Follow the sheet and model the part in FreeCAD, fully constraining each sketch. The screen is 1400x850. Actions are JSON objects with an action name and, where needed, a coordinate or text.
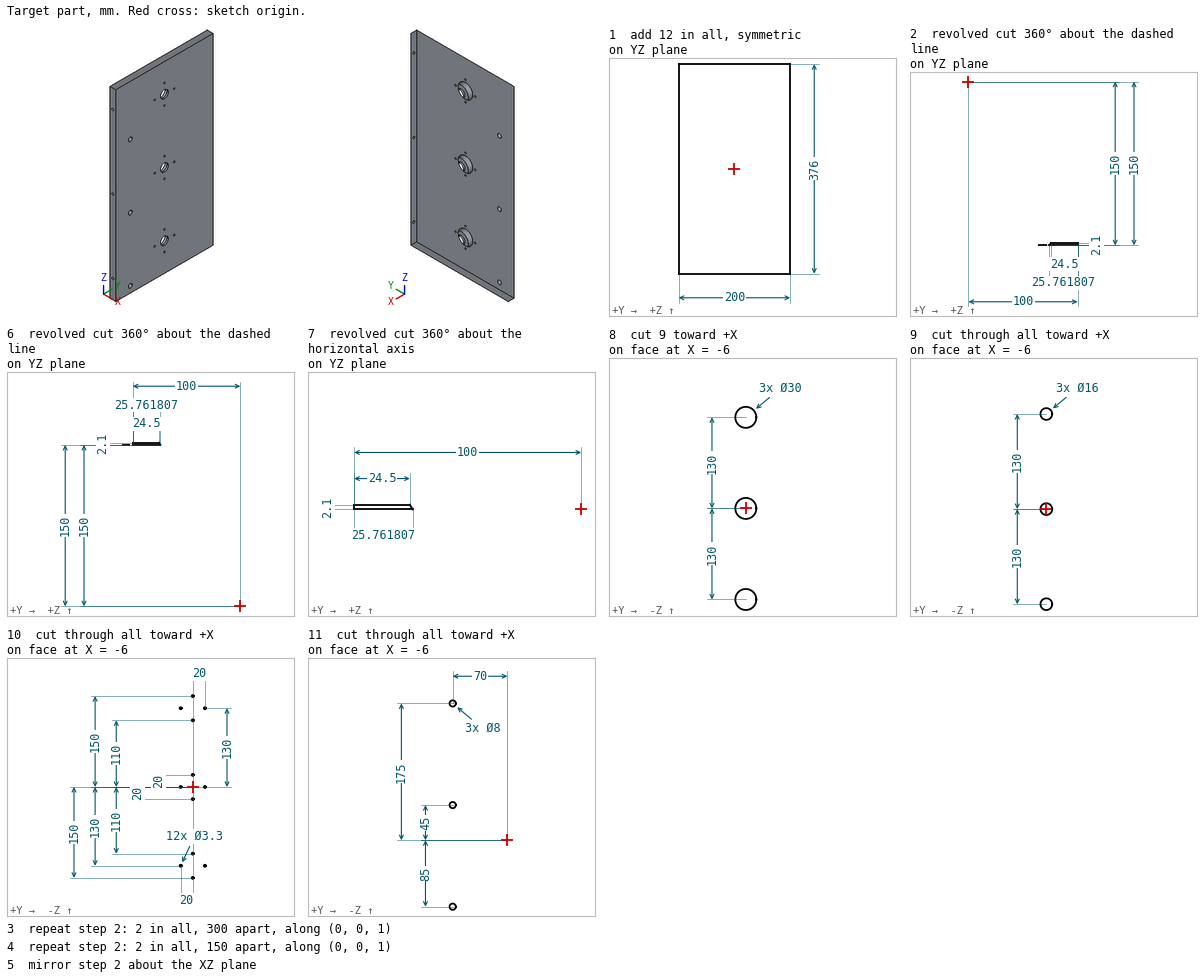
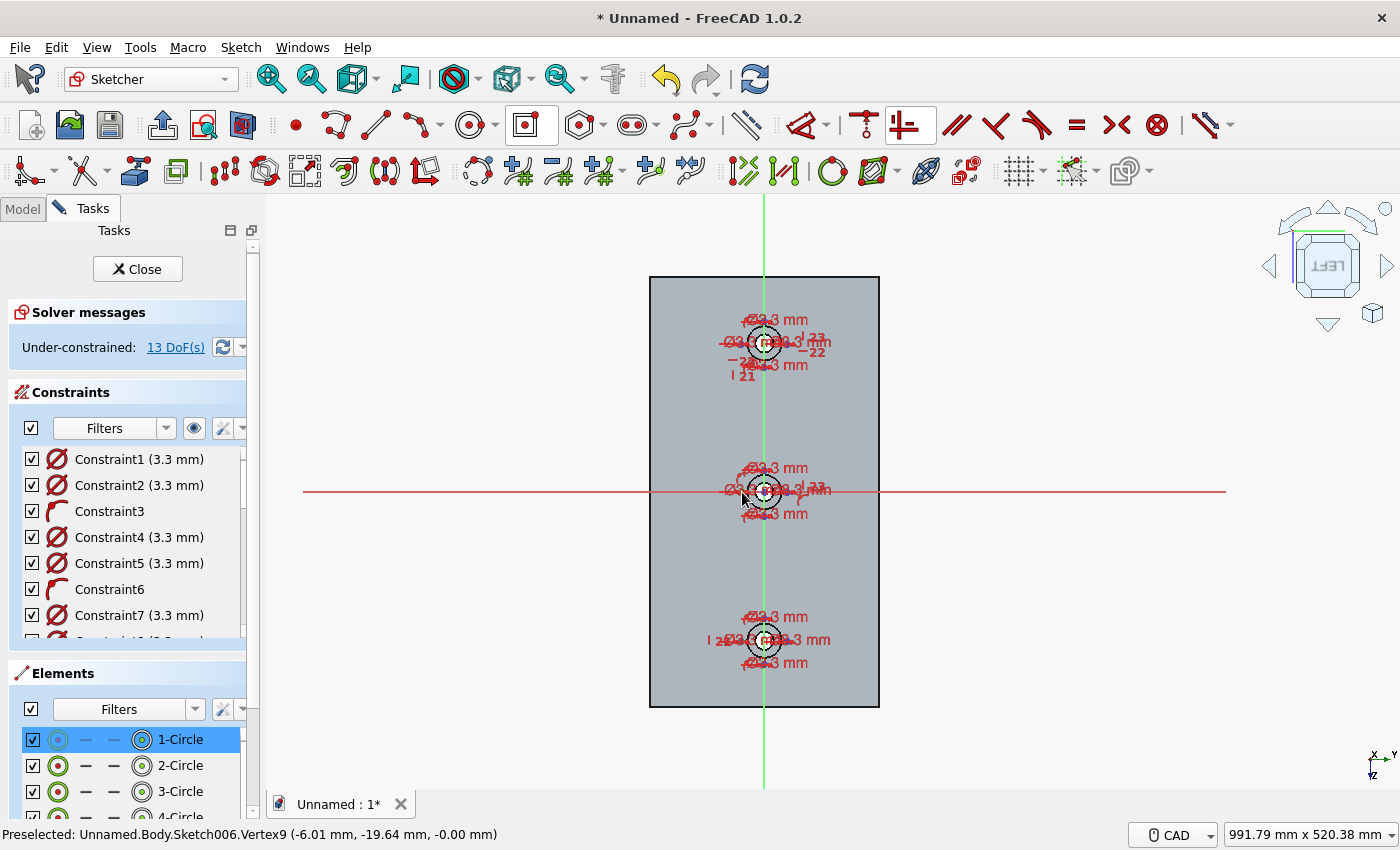
{"action": "key", "text": "v"}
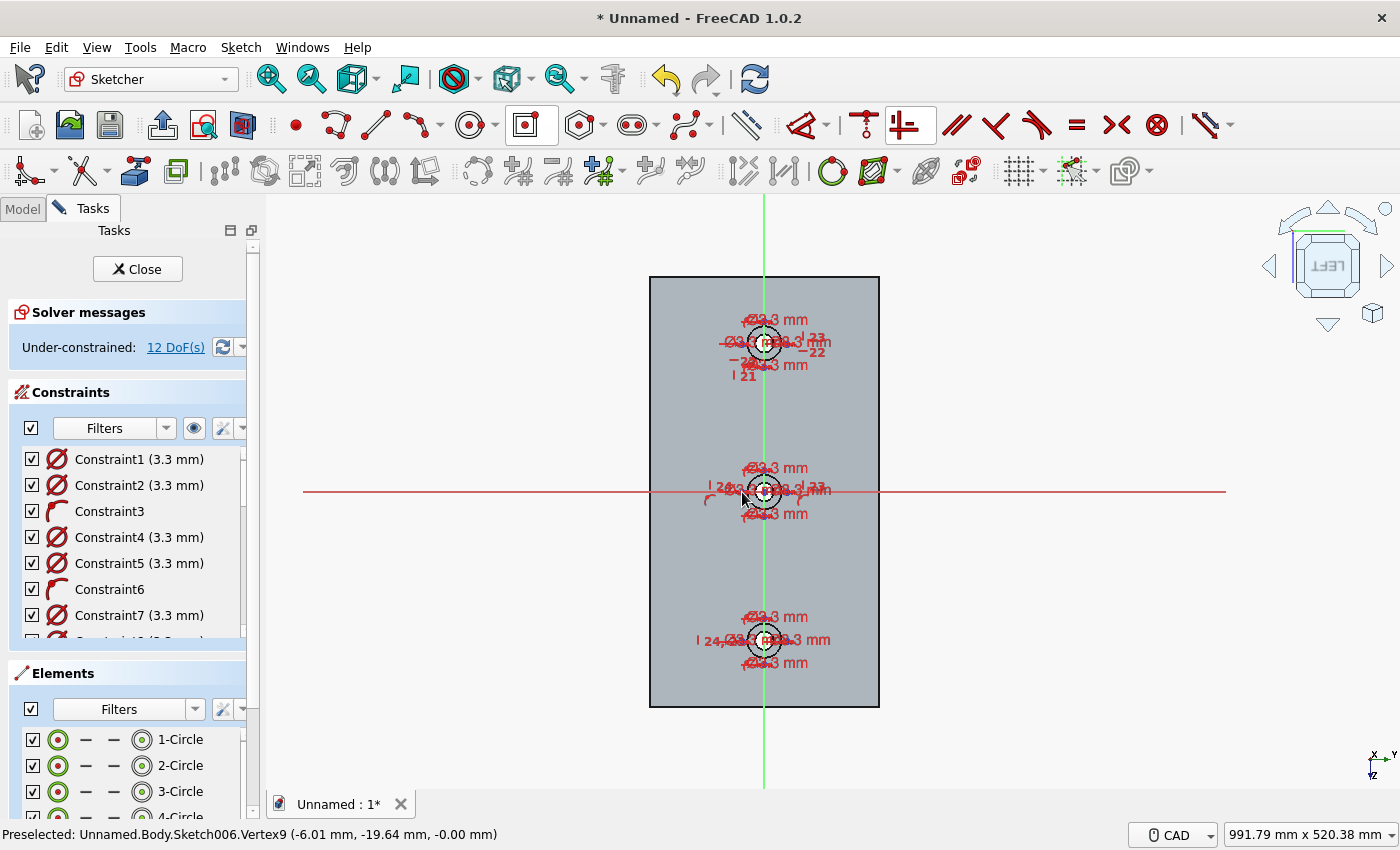
{"action": "left_click", "coordinate": [788, 492]}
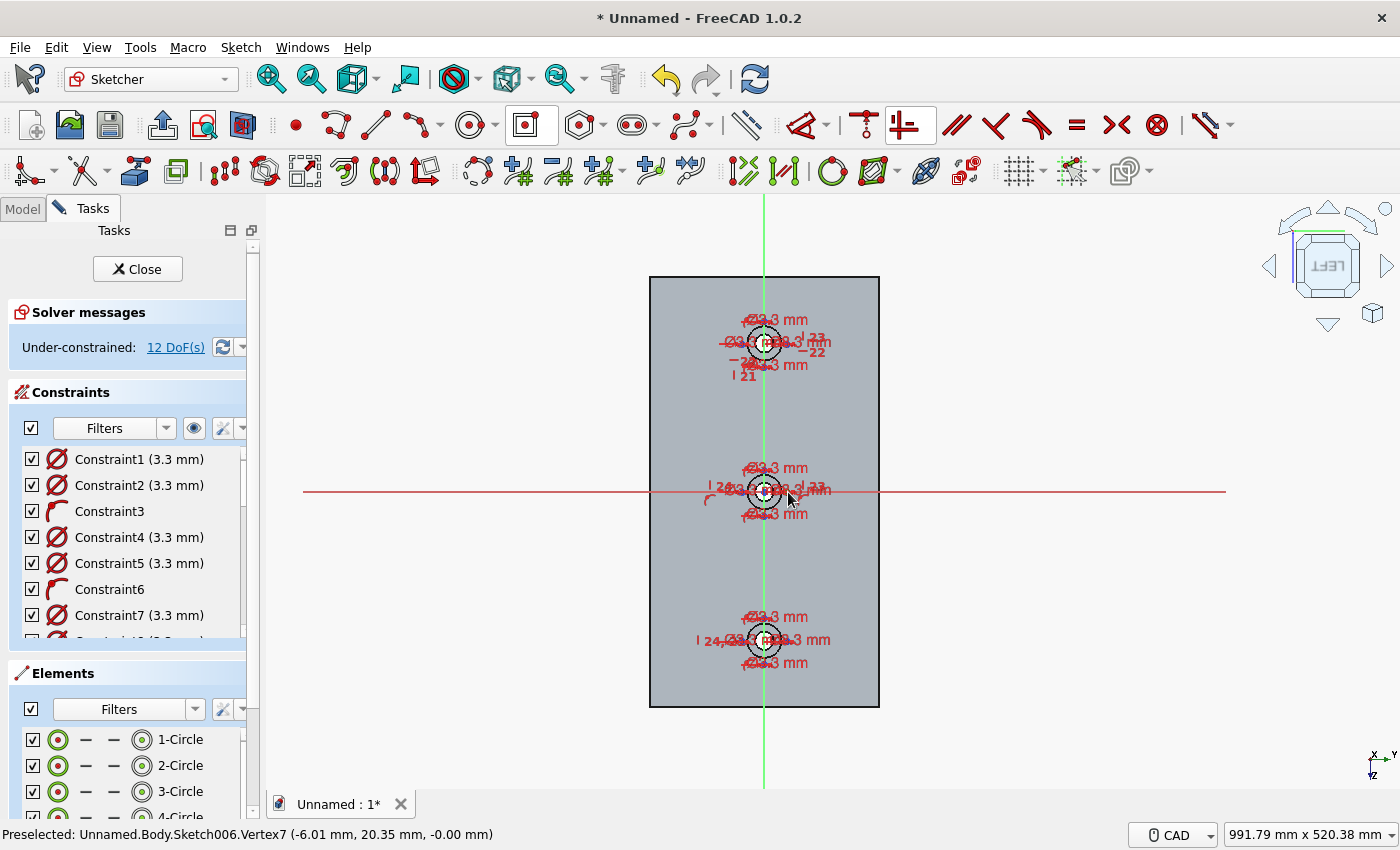
{"action": "left_click", "coordinate": [787, 642]}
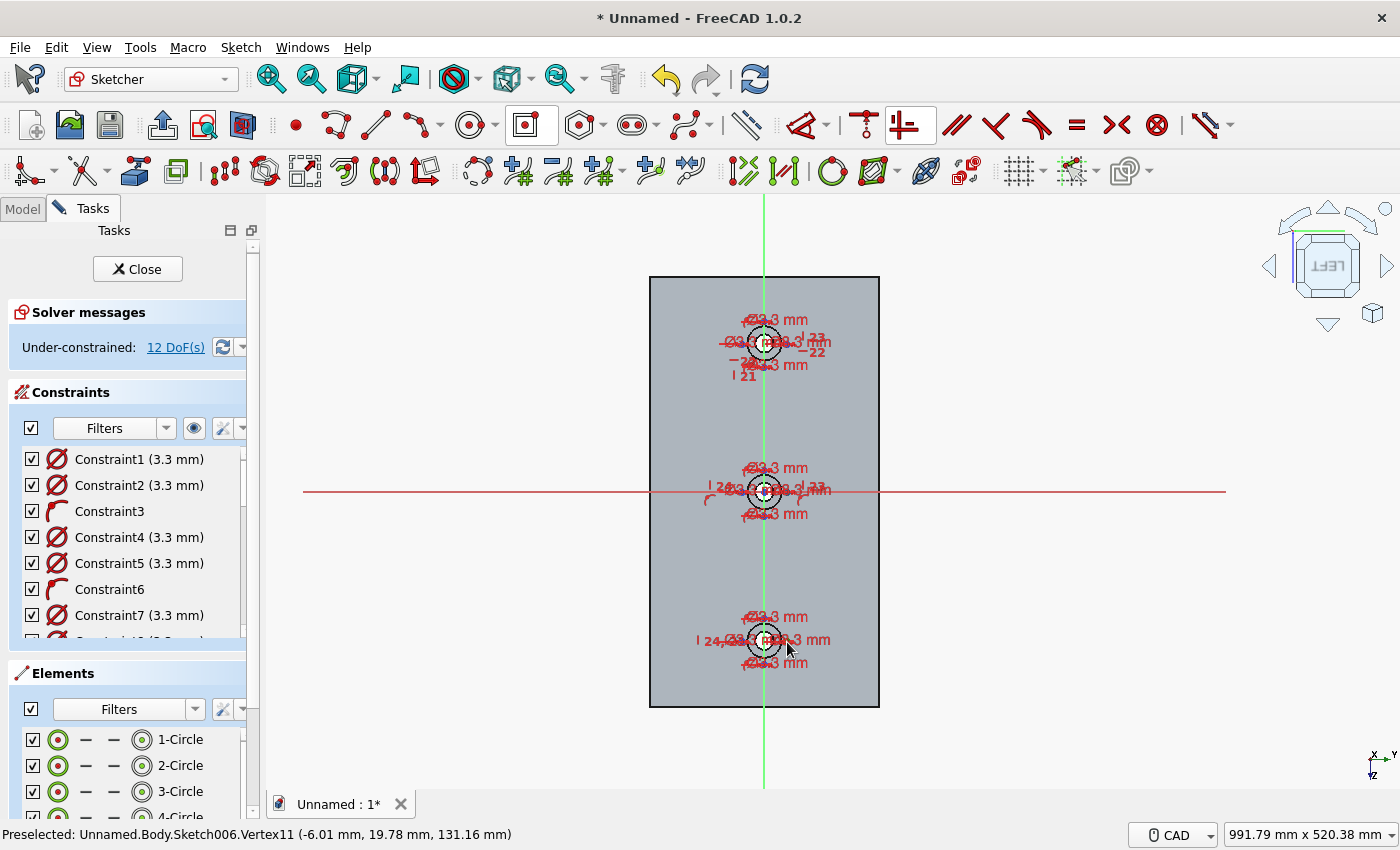
{"action": "key", "text": "v"}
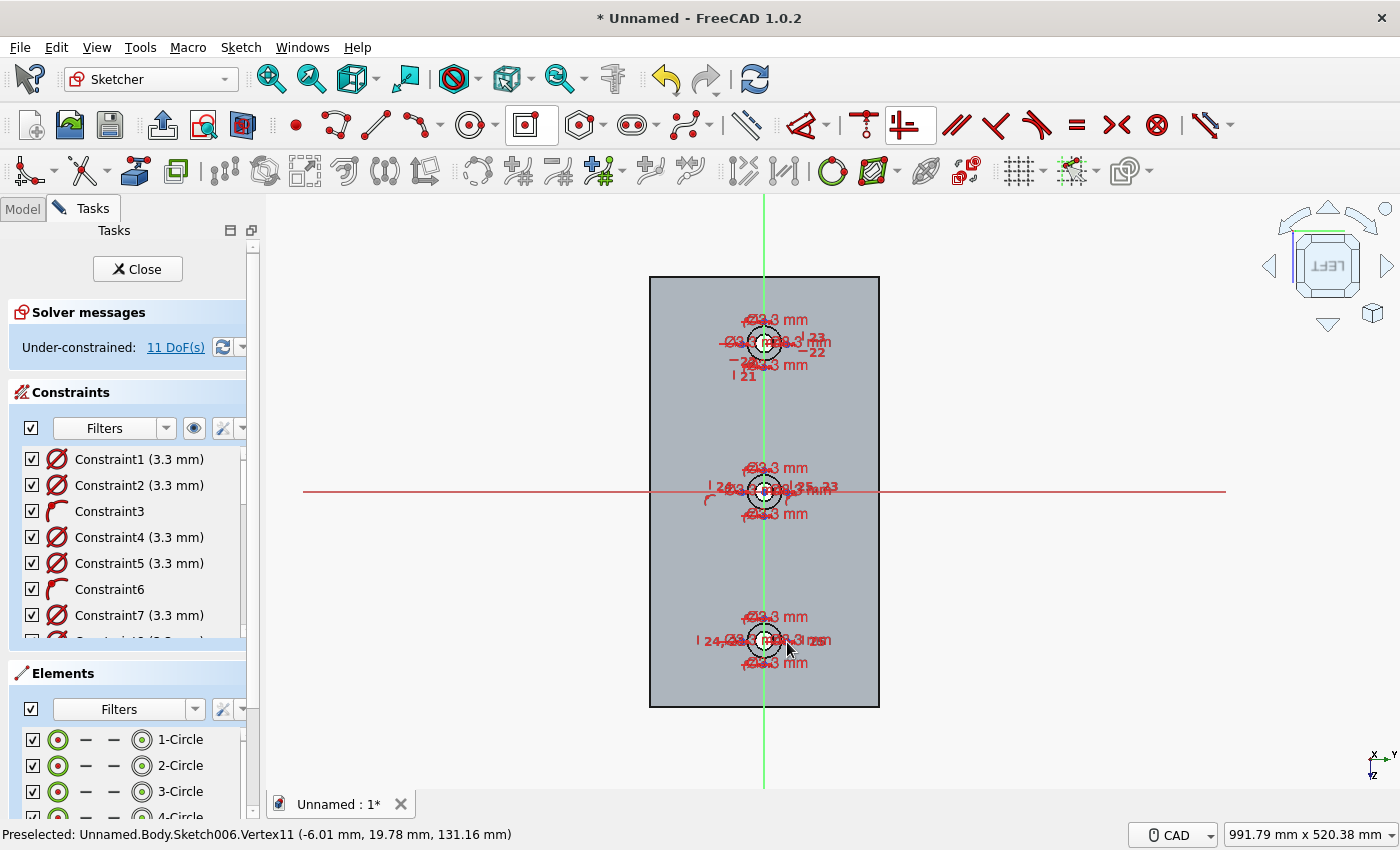
{"action": "left_click", "coordinate": [742, 642]}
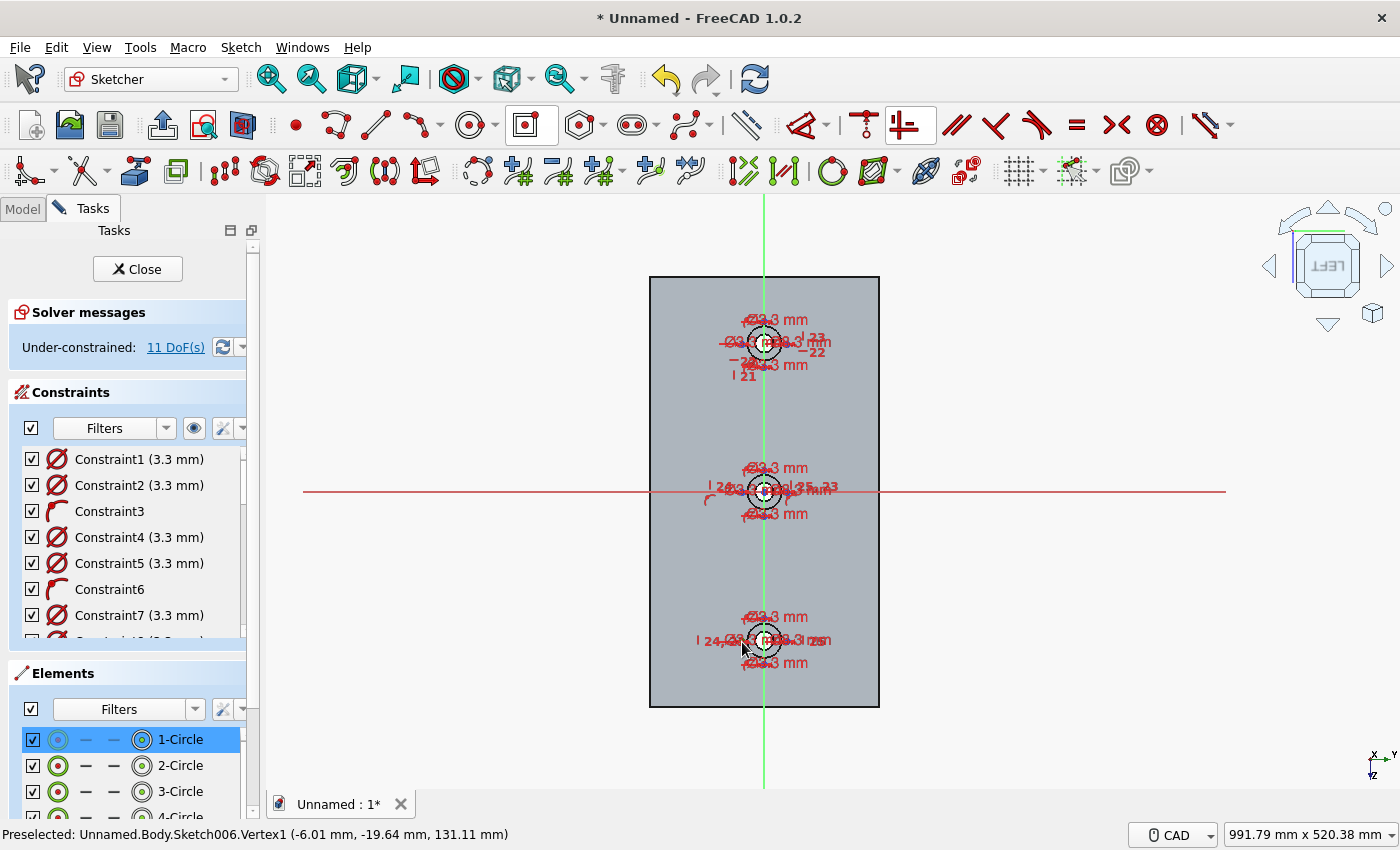
{"action": "left_click", "coordinate": [788, 642]}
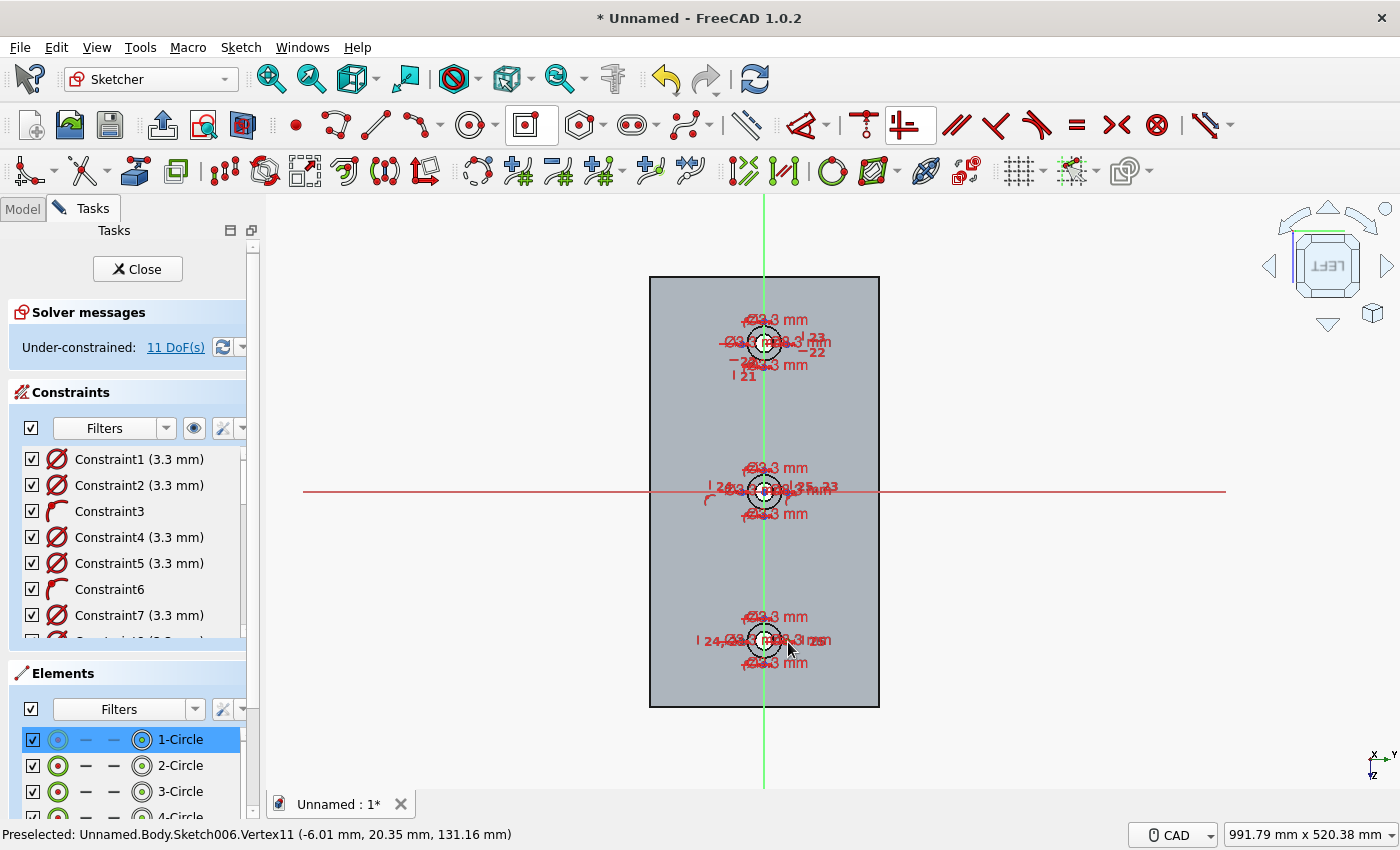
{"action": "key", "text": "h"}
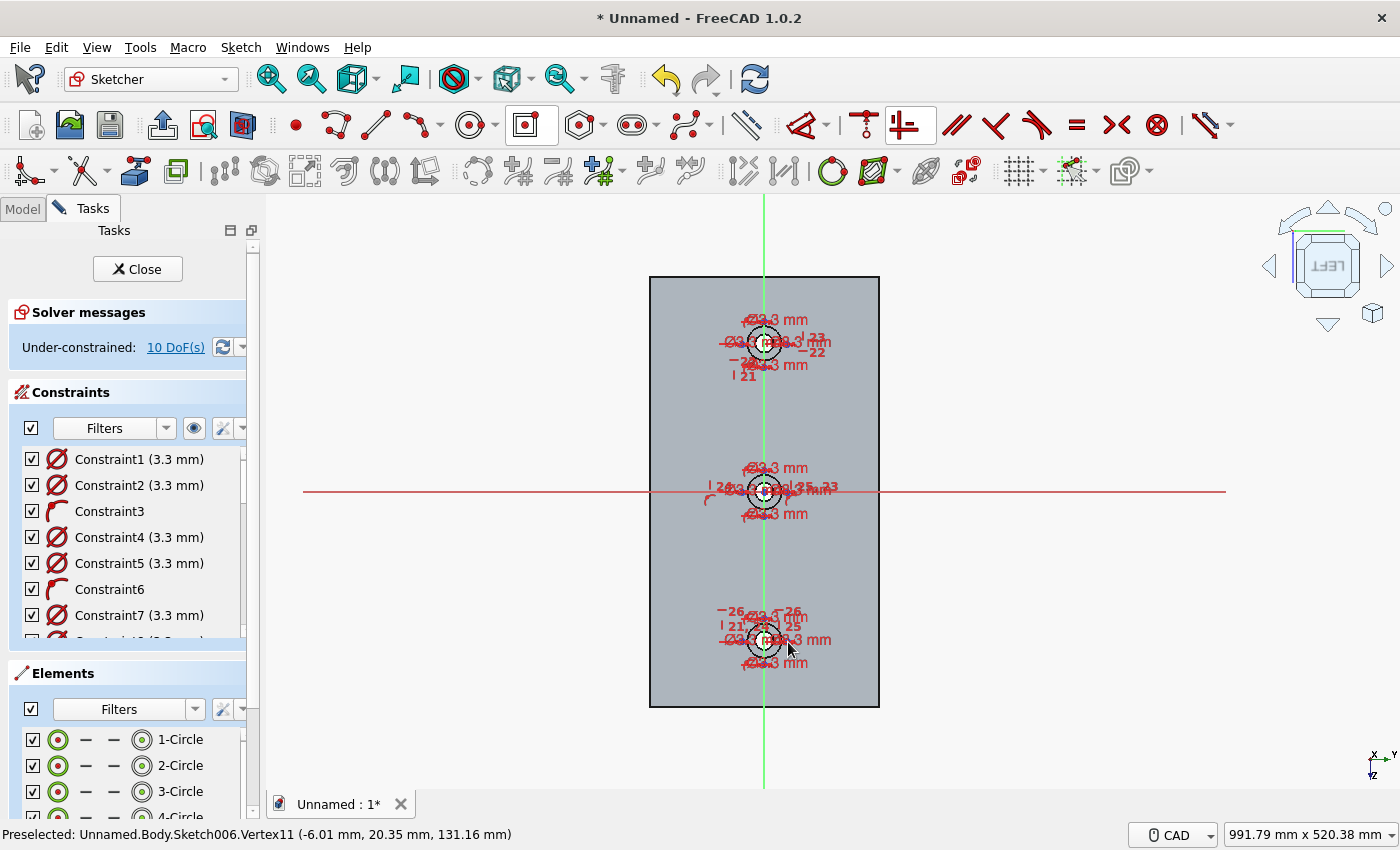
{"action": "left_click", "coordinate": [802, 126]}